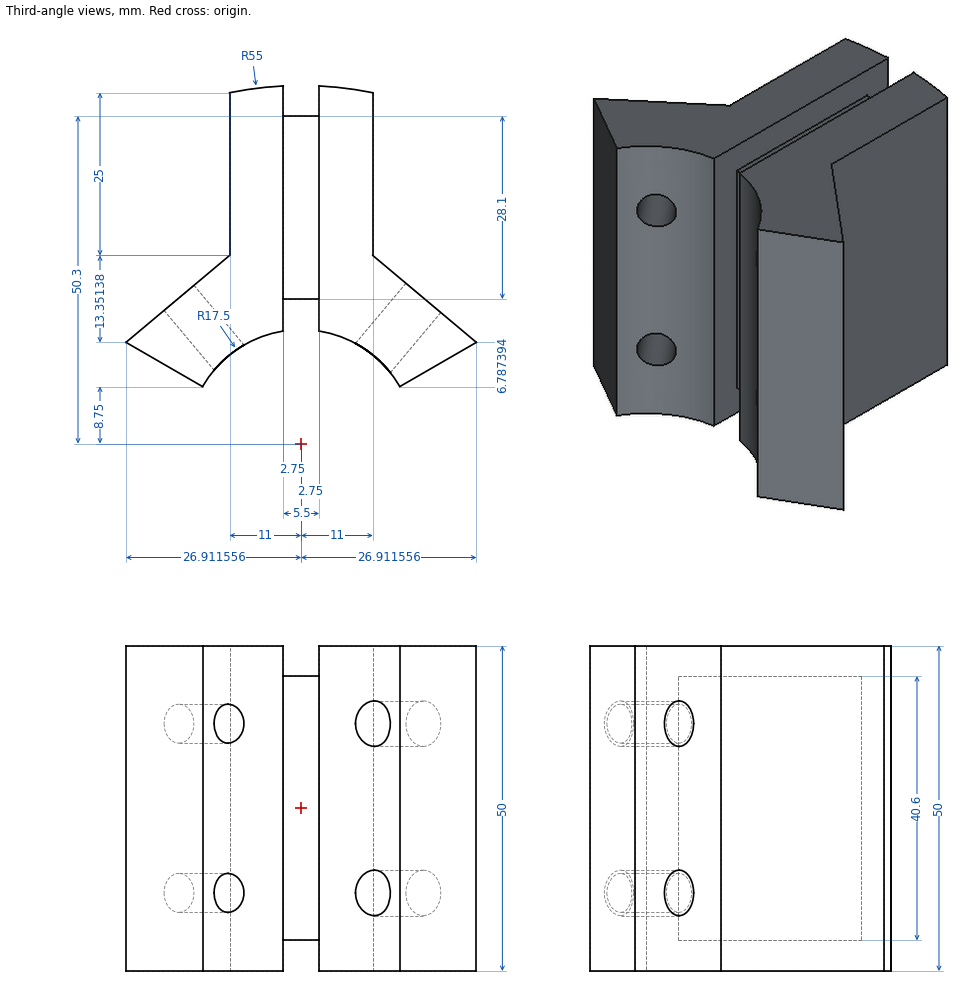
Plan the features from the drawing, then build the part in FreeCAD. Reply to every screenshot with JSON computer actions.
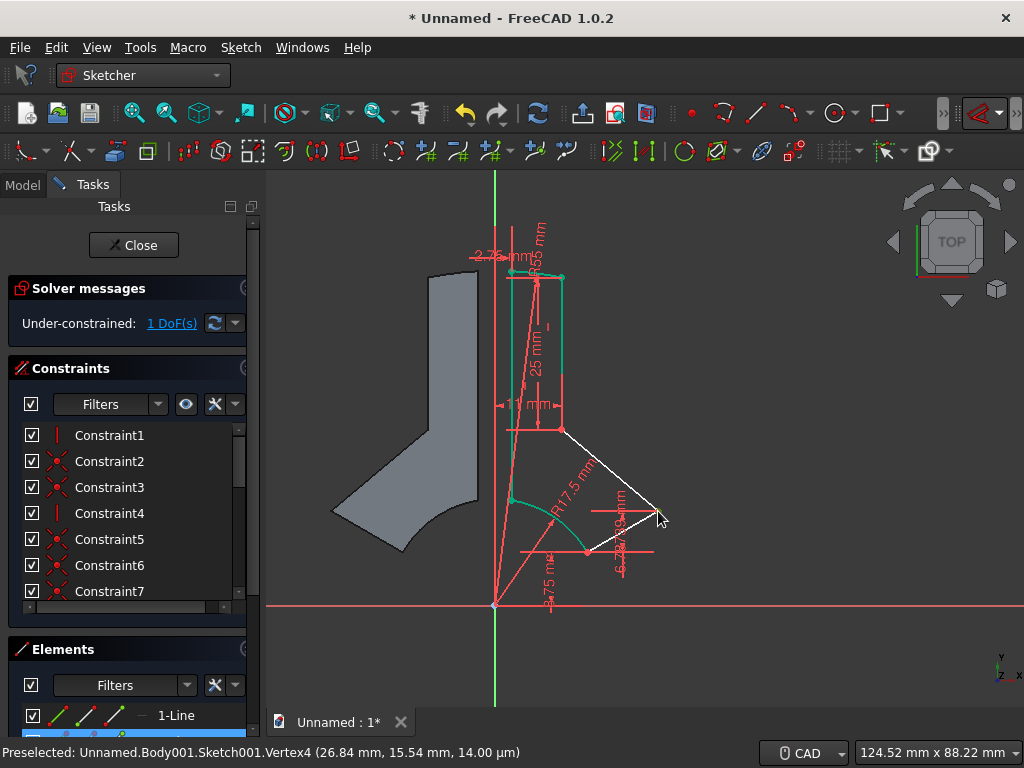
{"action": "left_click", "coordinate": [1002, 114]}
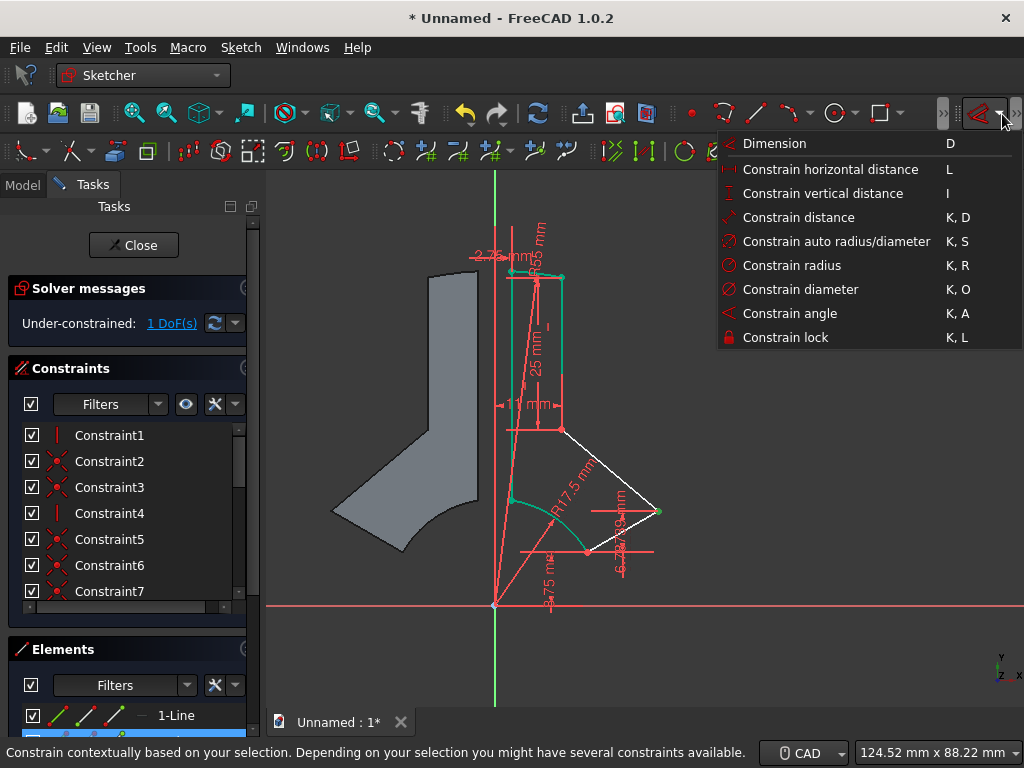
{"action": "left_click", "coordinate": [870, 169]}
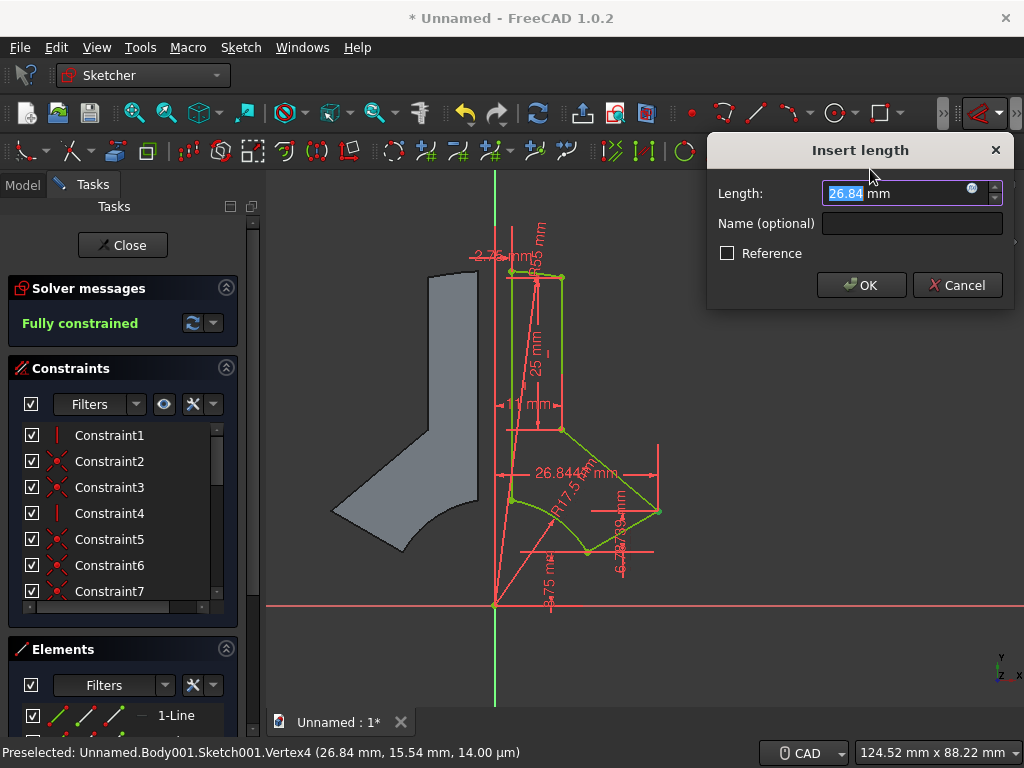
{"action": "type", "text": "26.911556"}
{"action": "key", "text": "Return"}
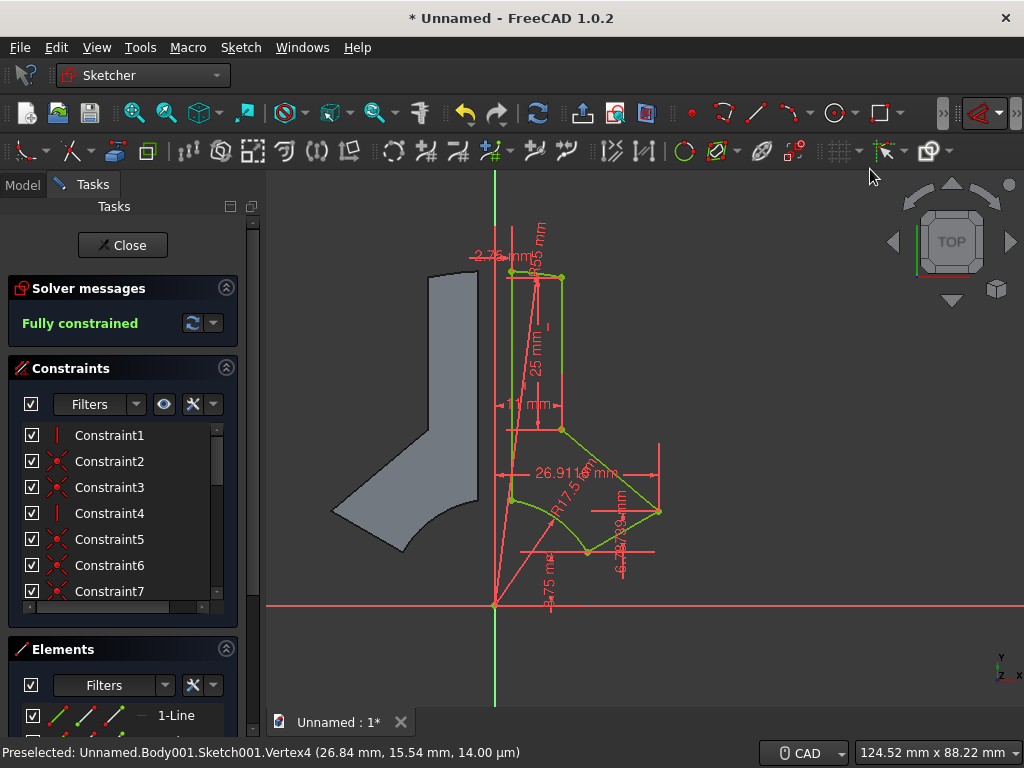
{"action": "left_click", "coordinate": [123, 245]}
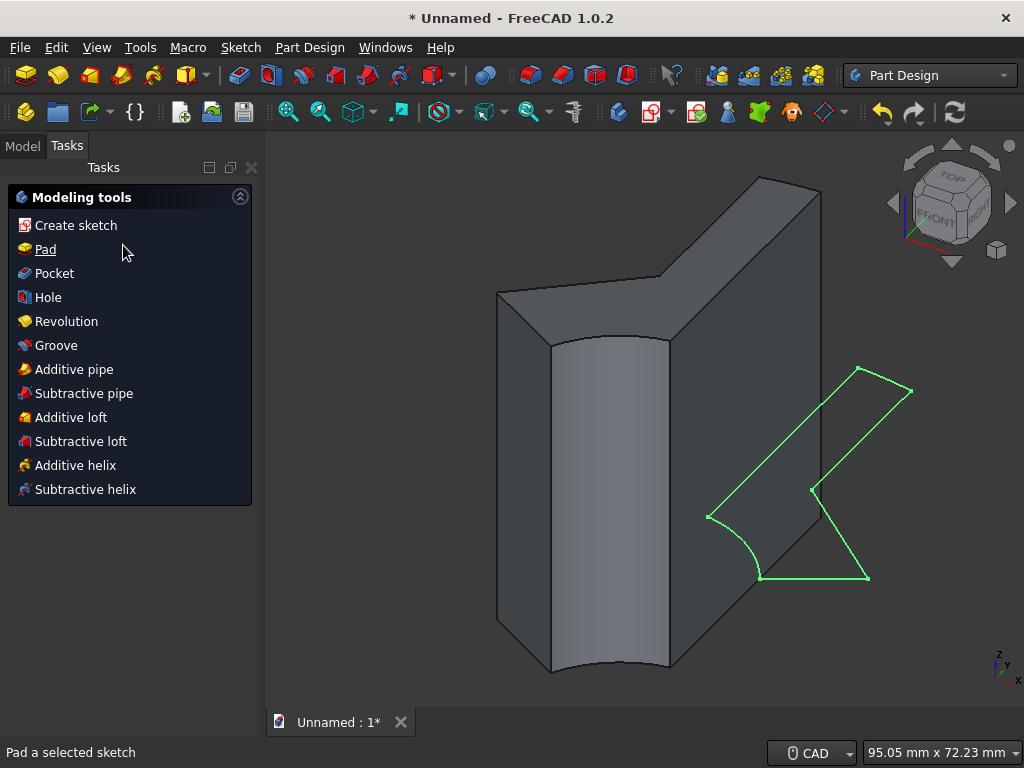
{"action": "left_click", "coordinate": [26, 76]}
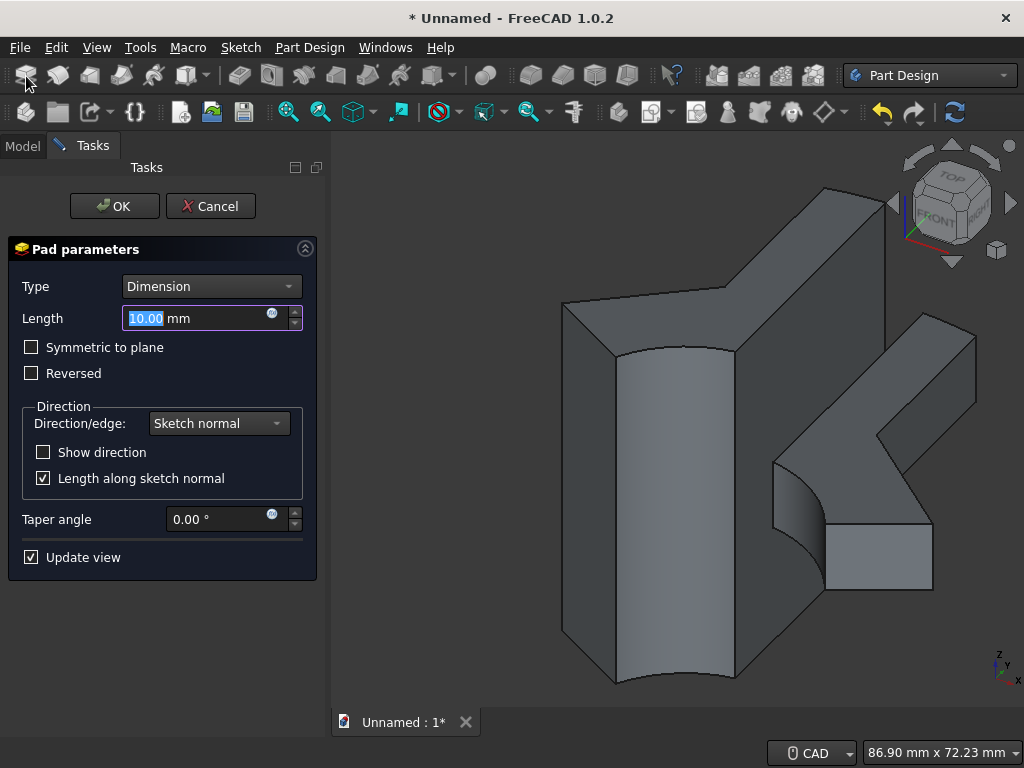
{"action": "type", "text": "50"}
{"action": "key", "text": "Tab"}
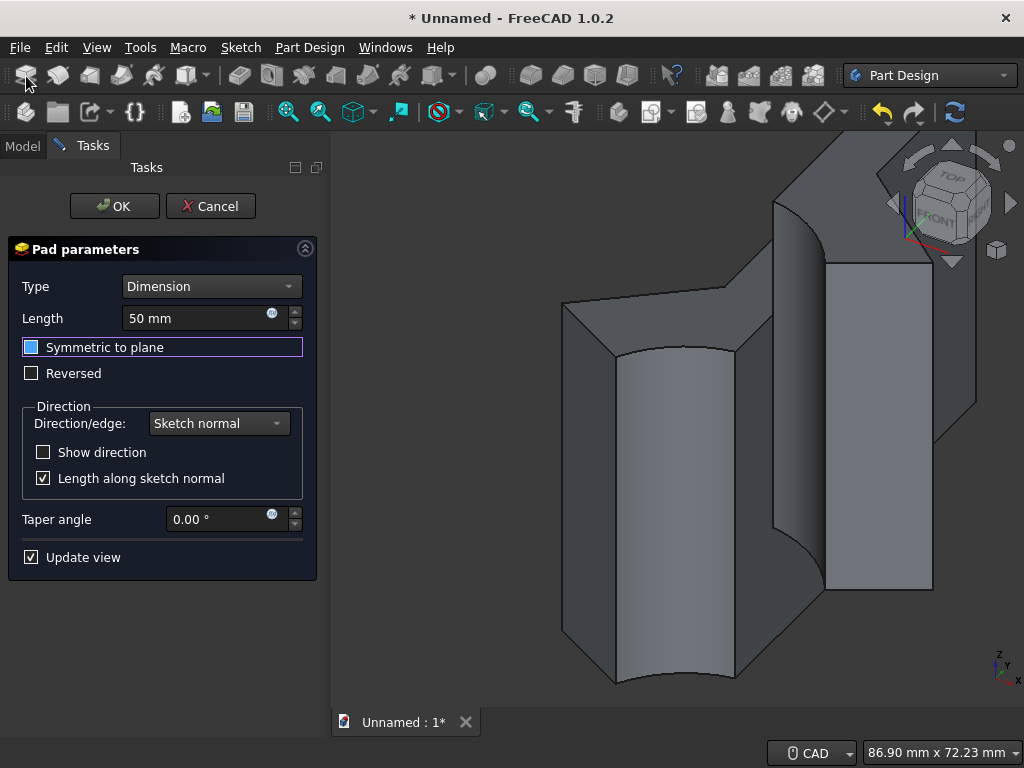
{"action": "left_click", "coordinate": [30, 347]}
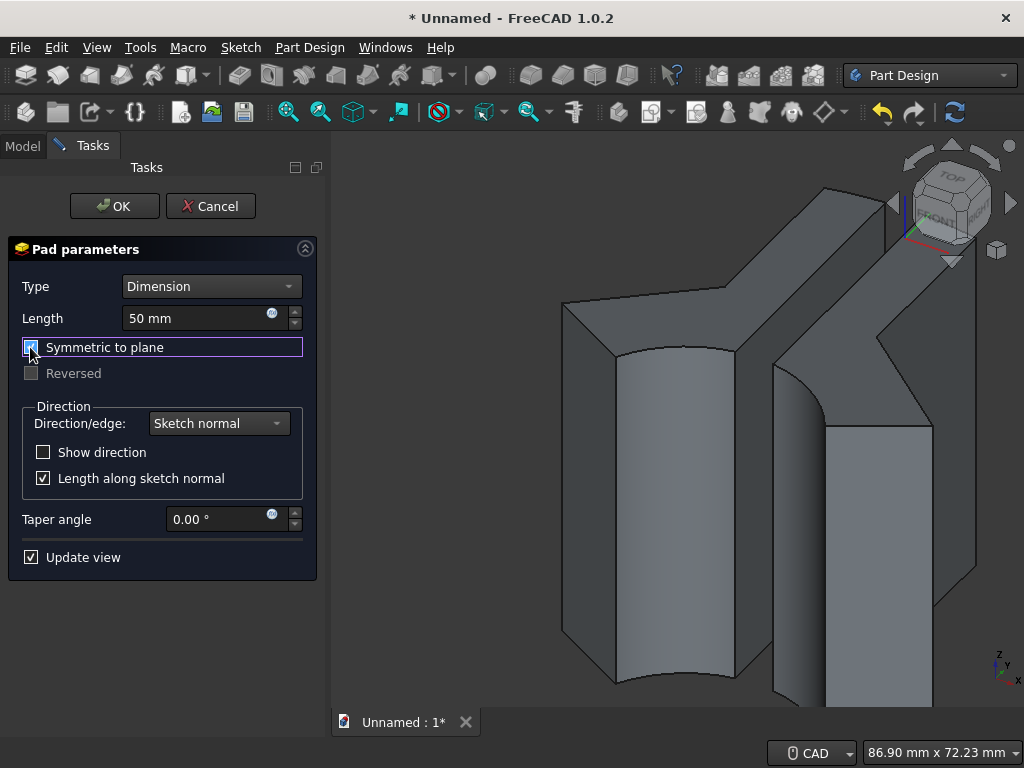
{"action": "left_click", "coordinate": [115, 206]}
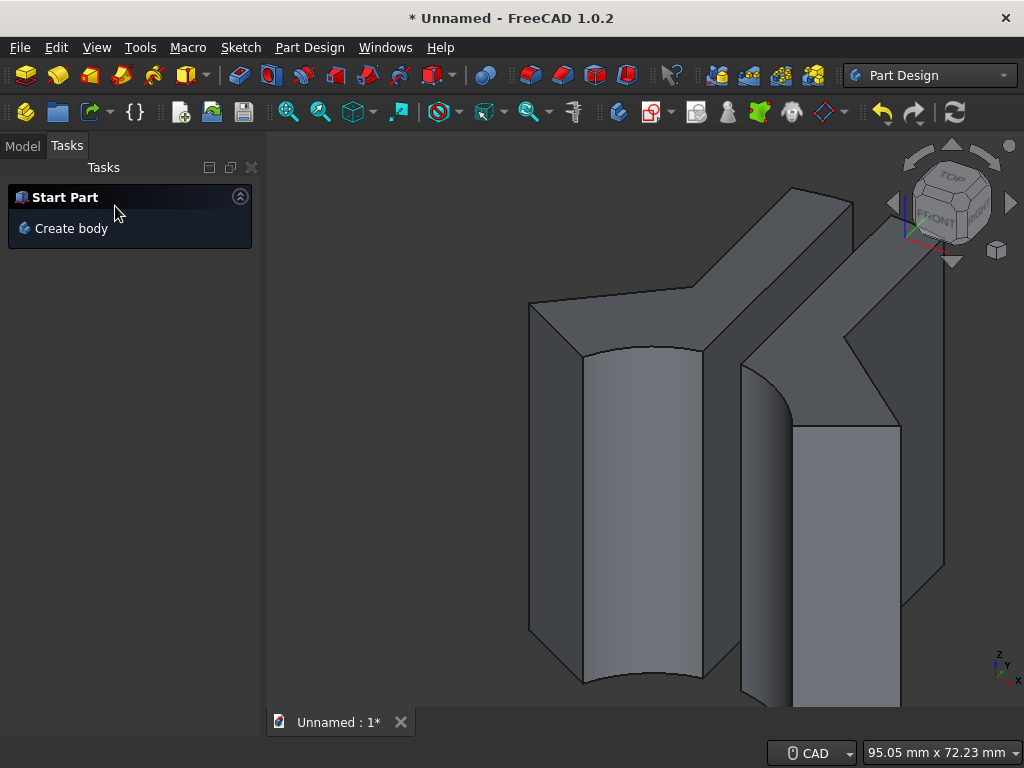
{"action": "left_click", "coordinate": [290, 112]}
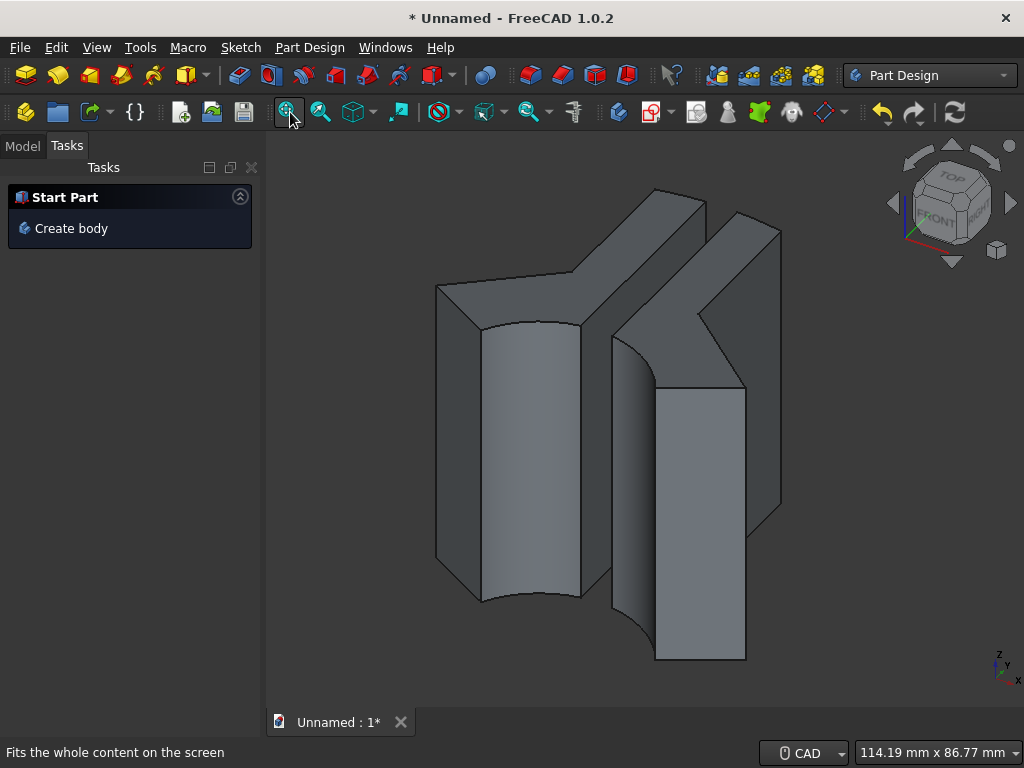
{"action": "left_click", "coordinate": [23, 145]}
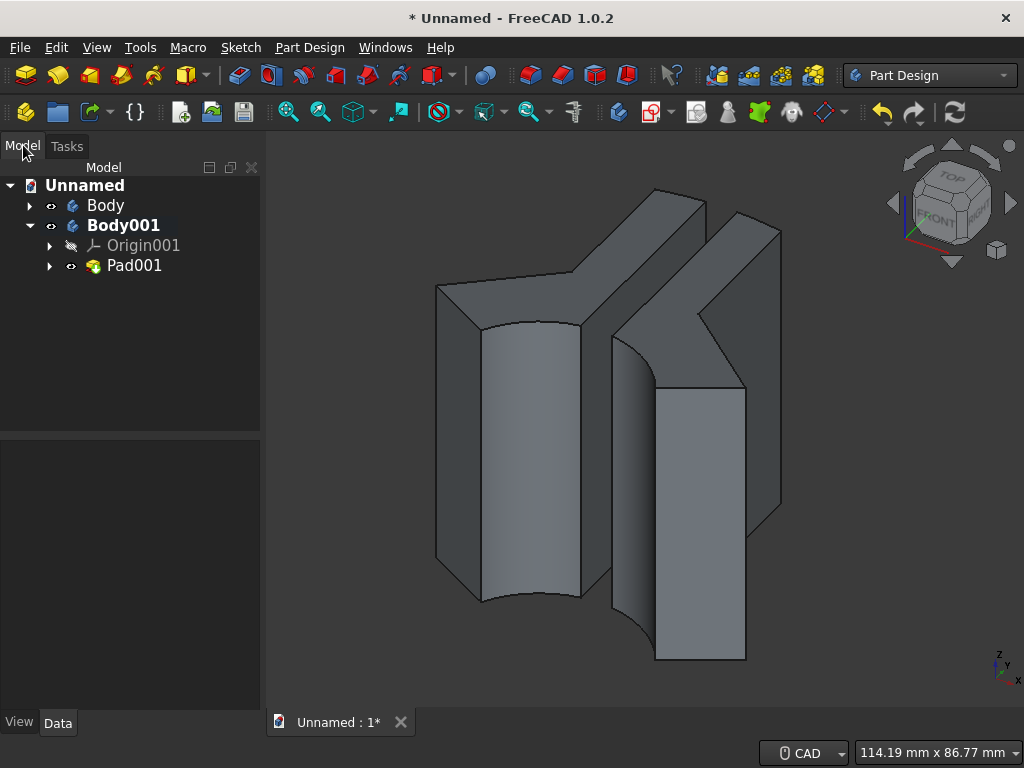
{"action": "double_click", "coordinate": [96, 206]}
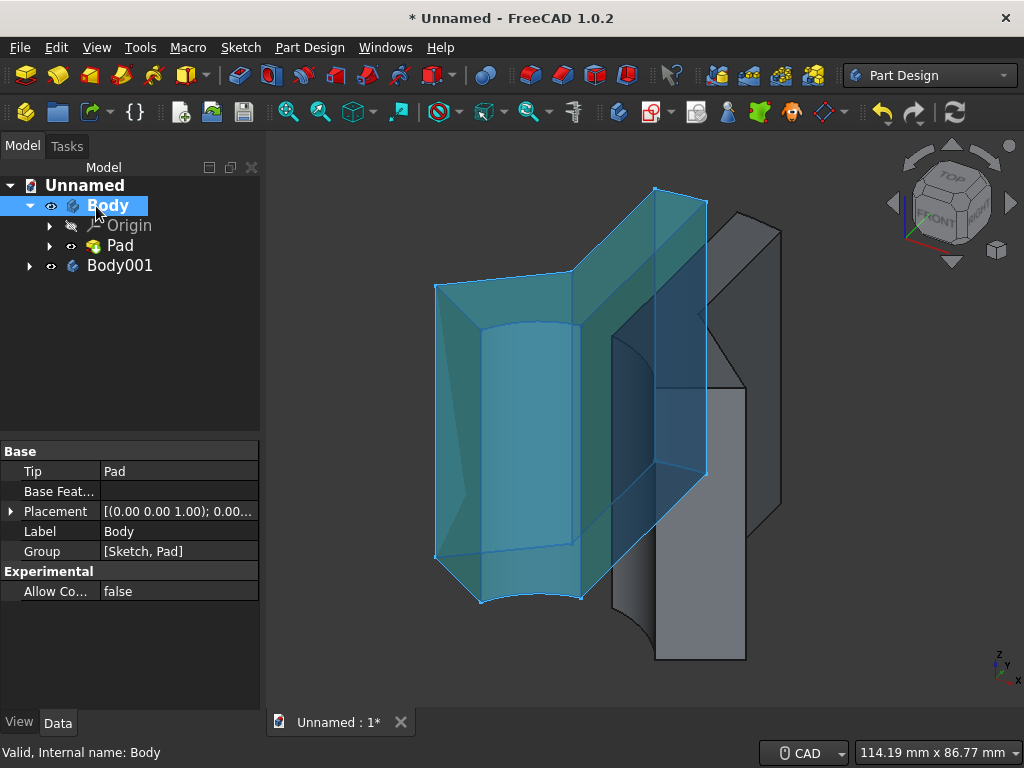
{"action": "left_click", "coordinate": [96, 206]}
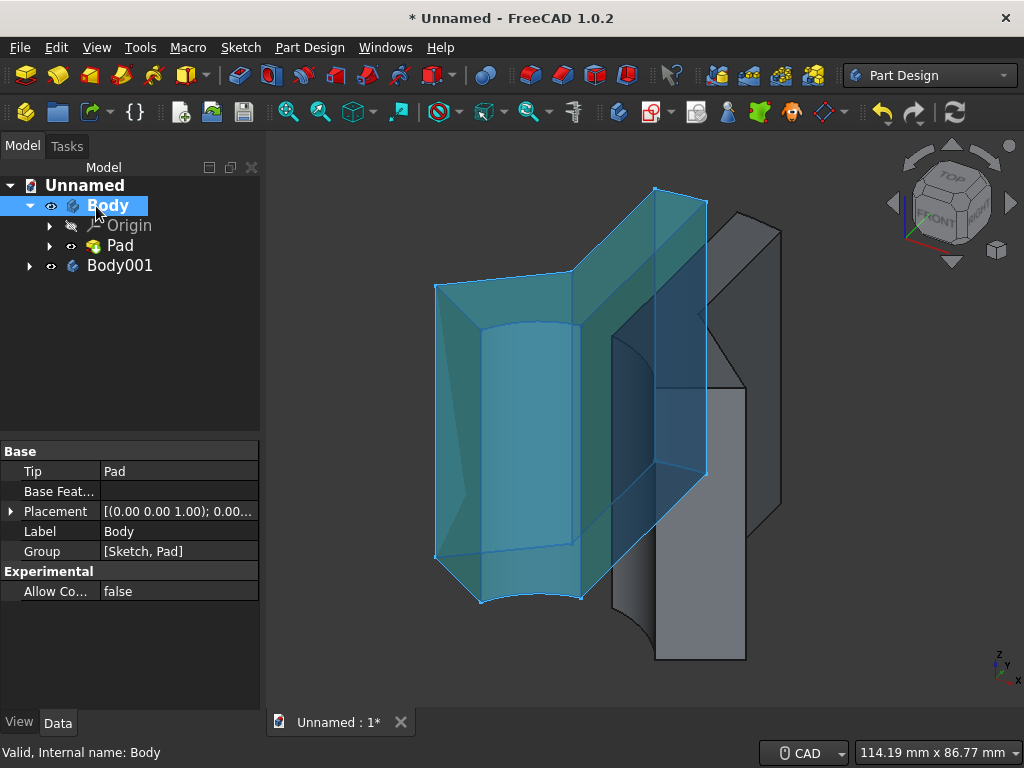
{"action": "left_click", "coordinate": [146, 591]}